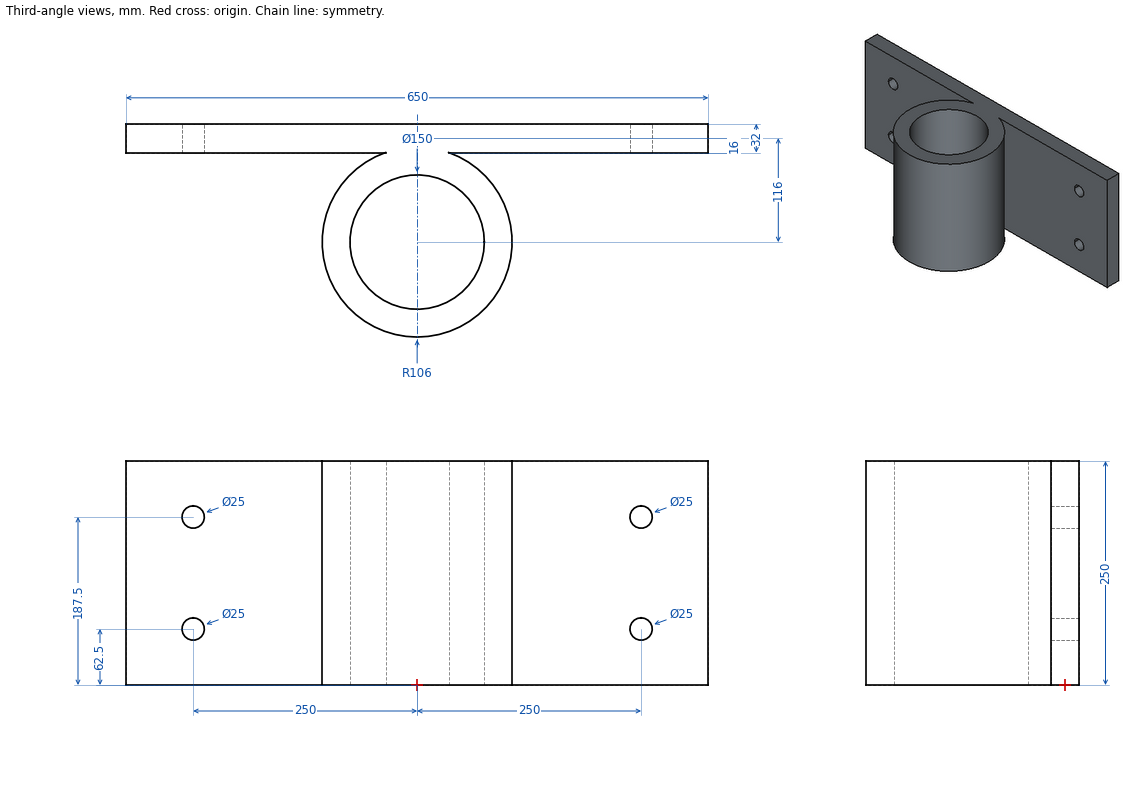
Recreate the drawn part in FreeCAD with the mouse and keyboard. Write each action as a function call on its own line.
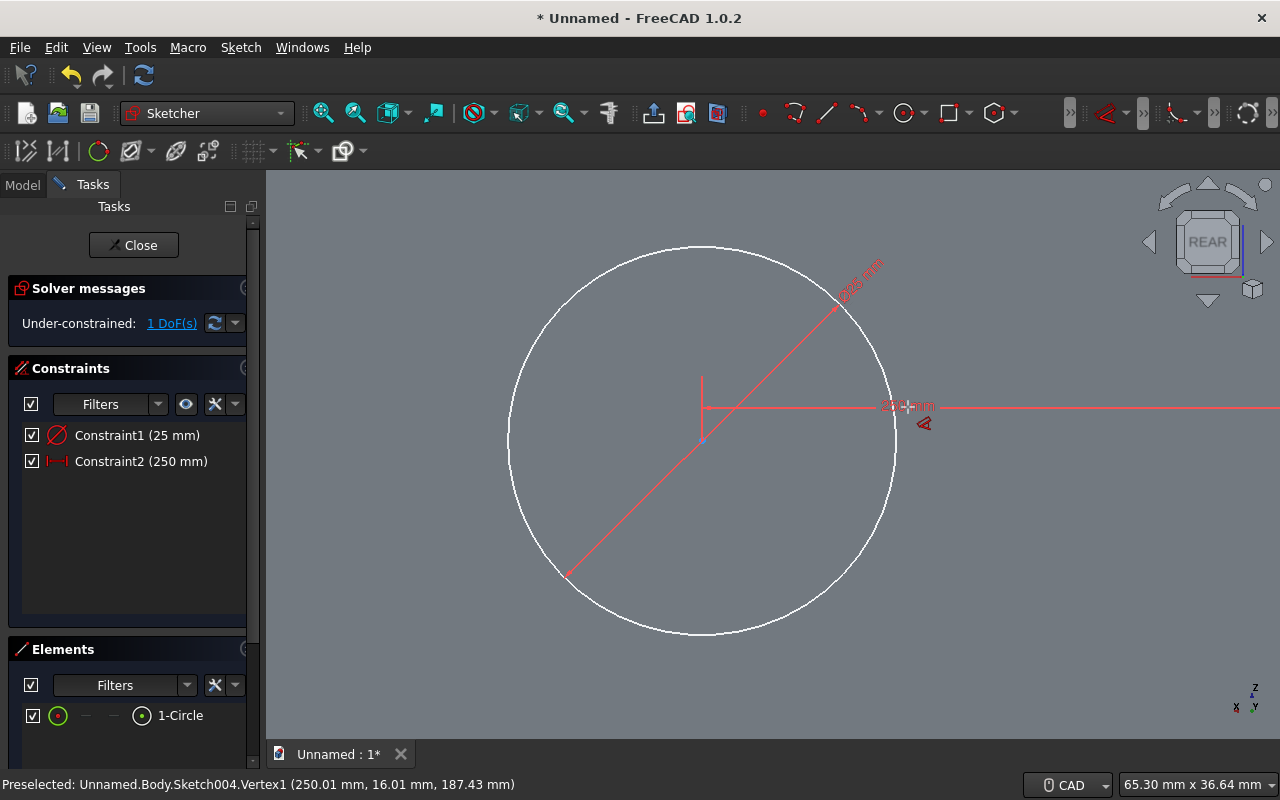
click(702, 441)
click(668, 576)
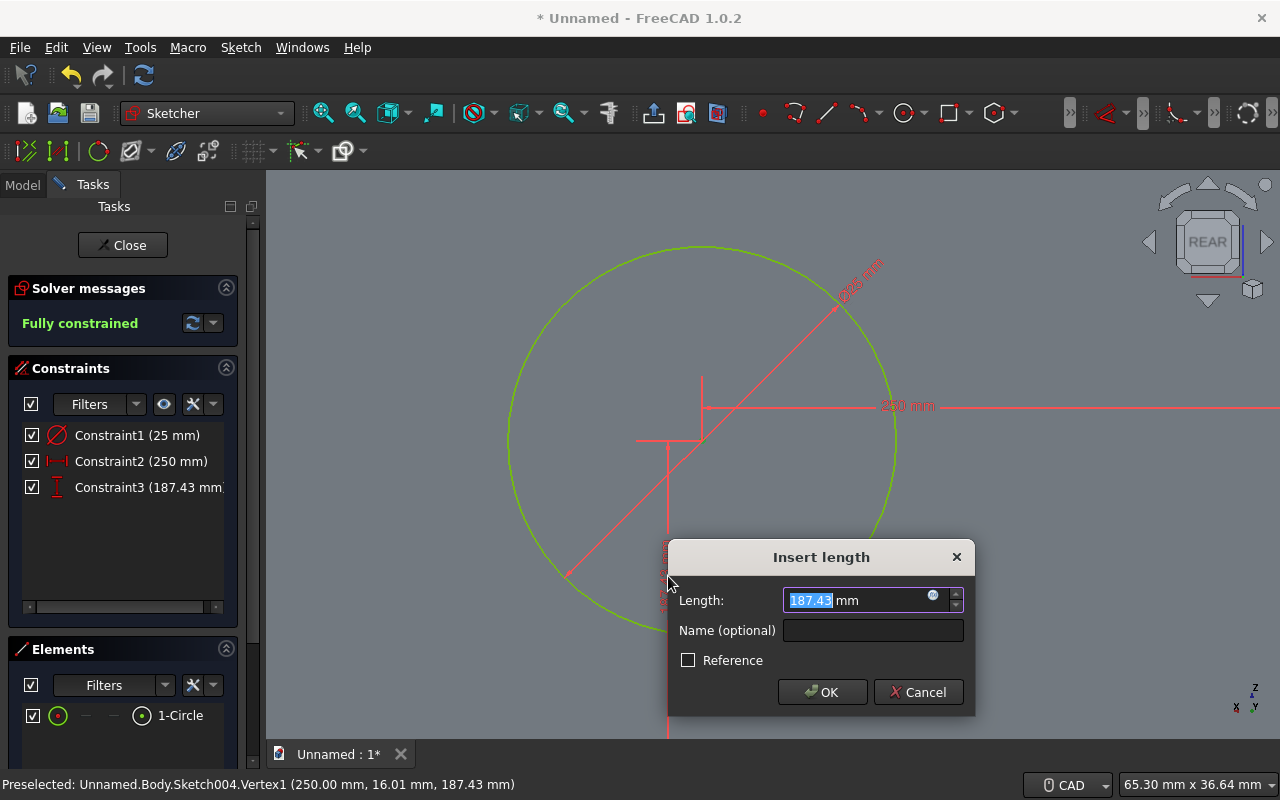
text(187.5)
key(Return)
key(Escape)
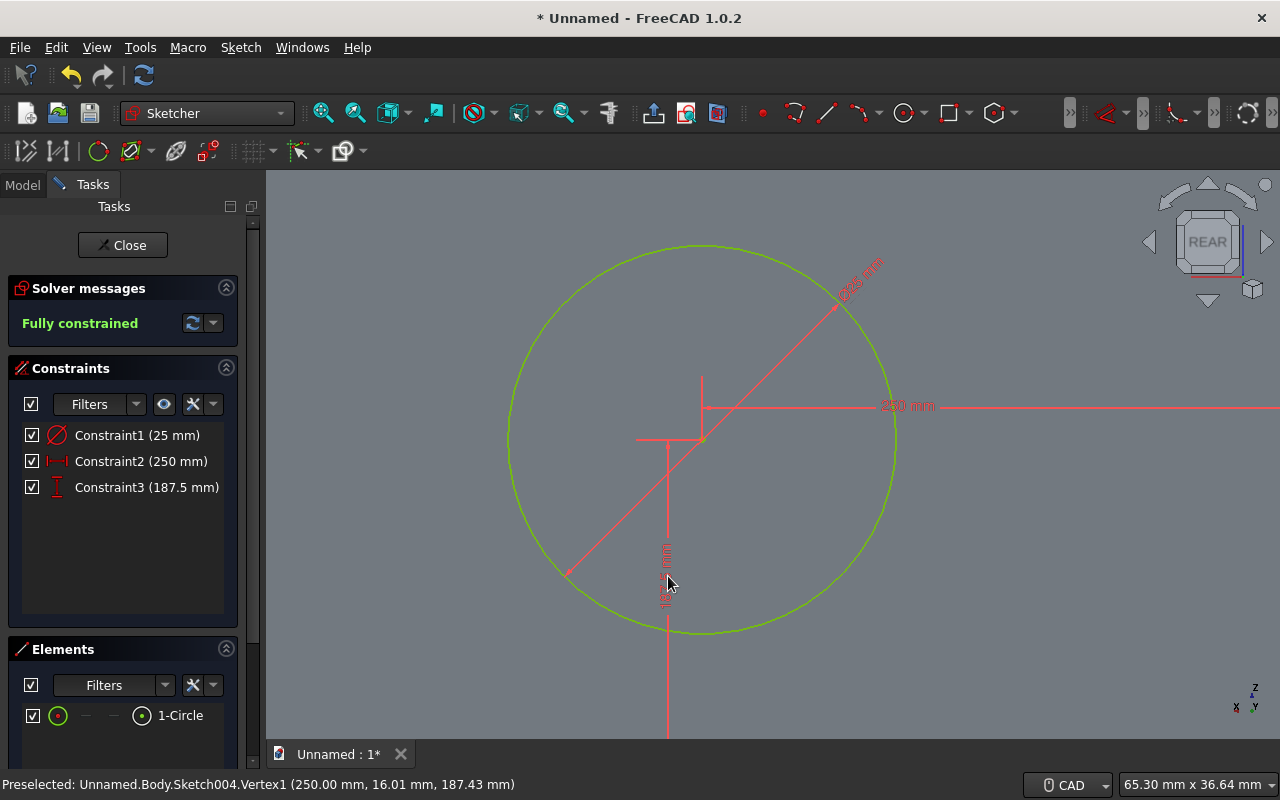
click(123, 245)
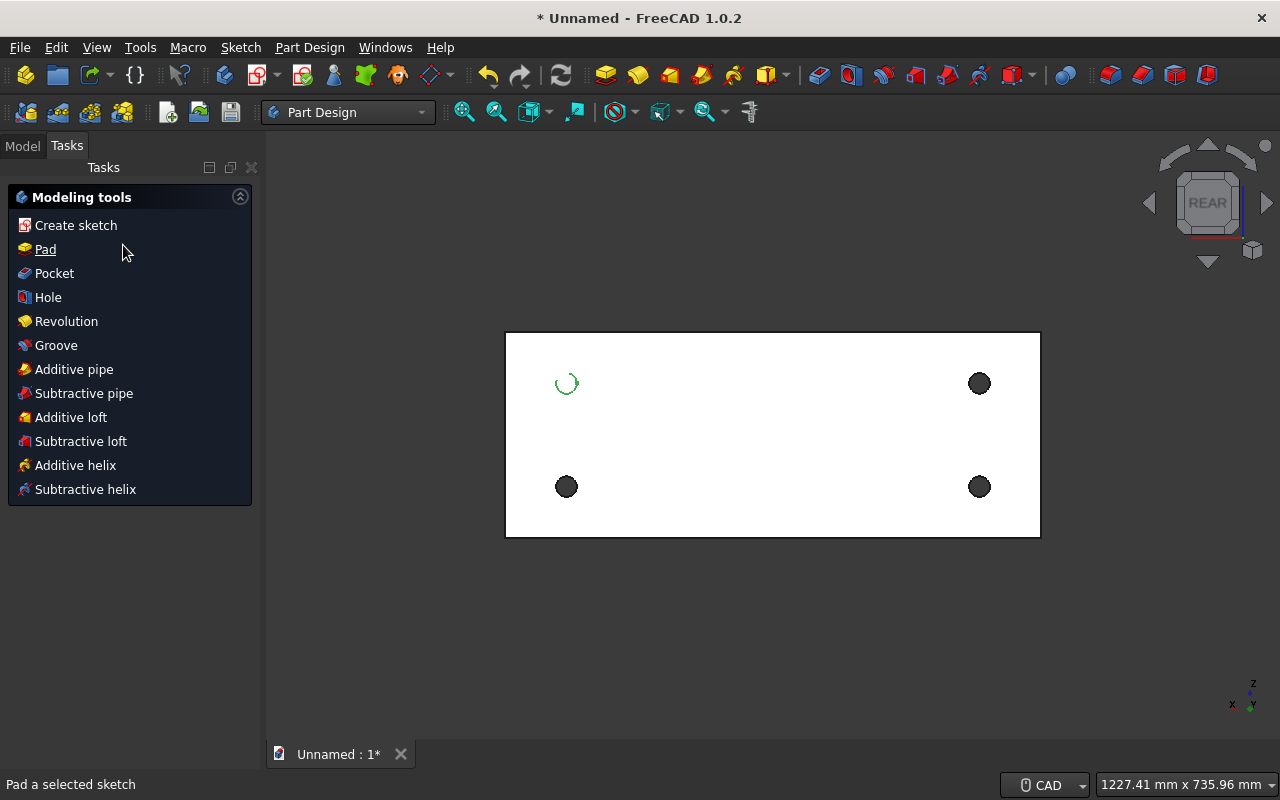
click(820, 76)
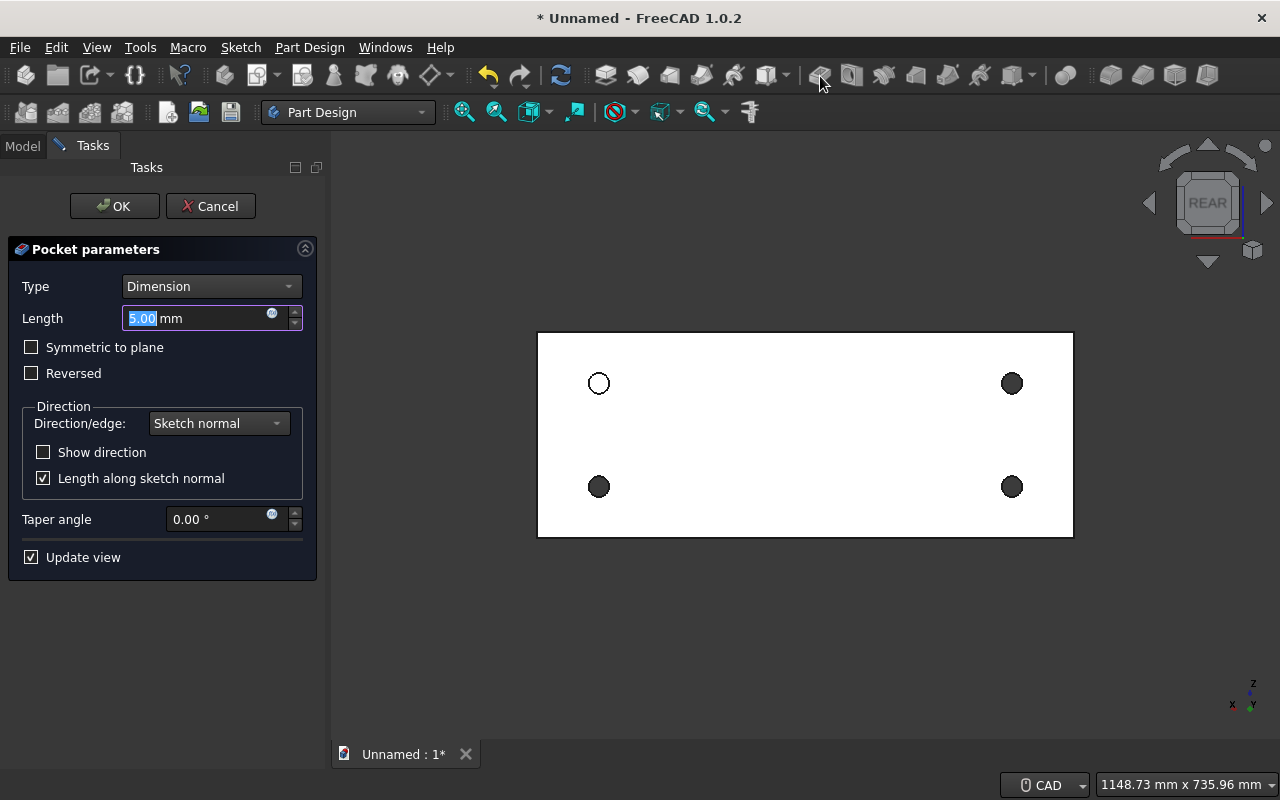
click(212, 286)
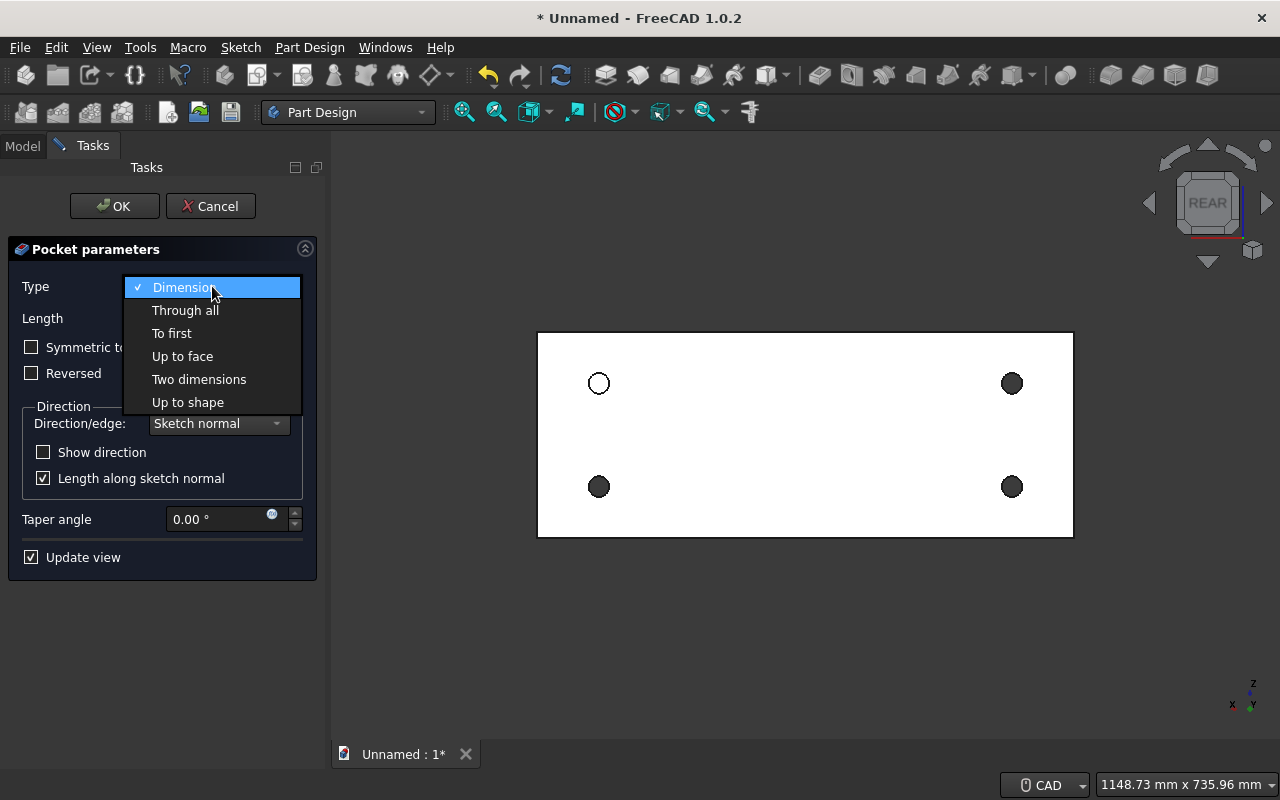
click(212, 334)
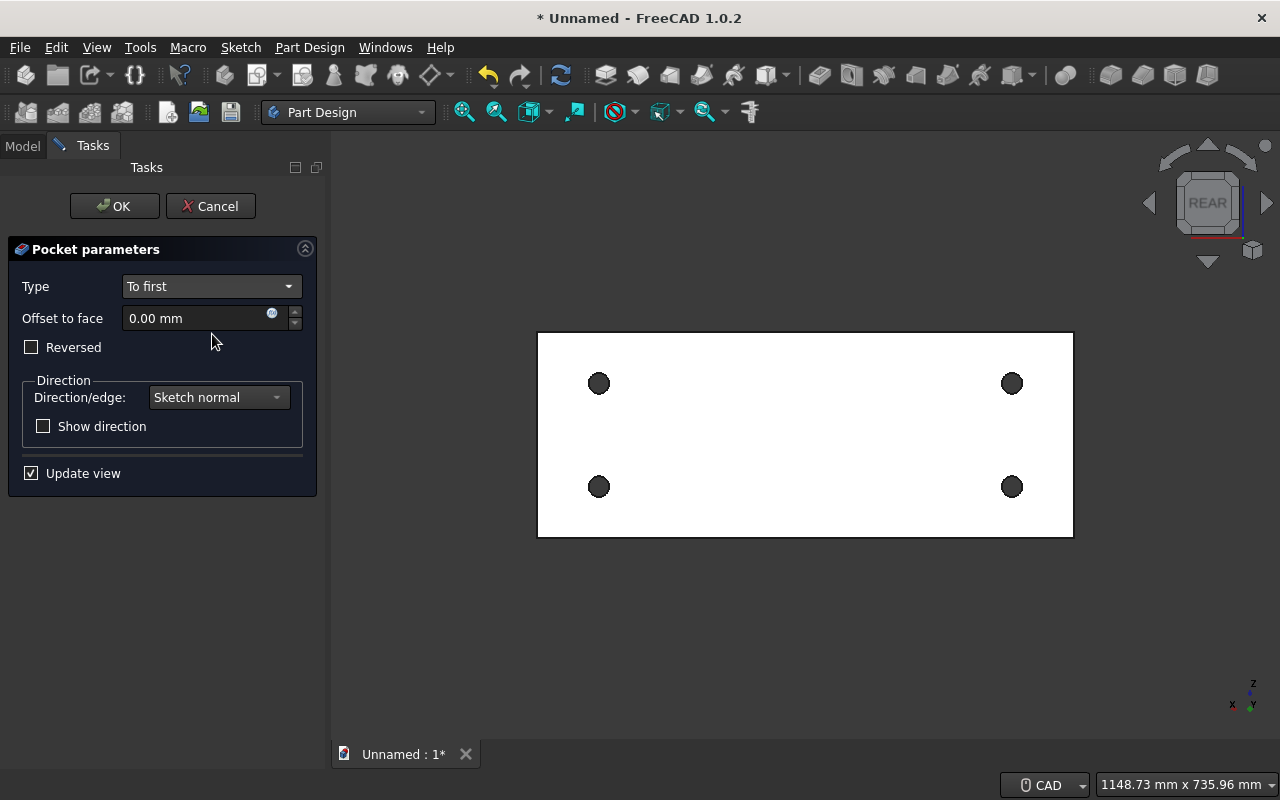
click(115, 206)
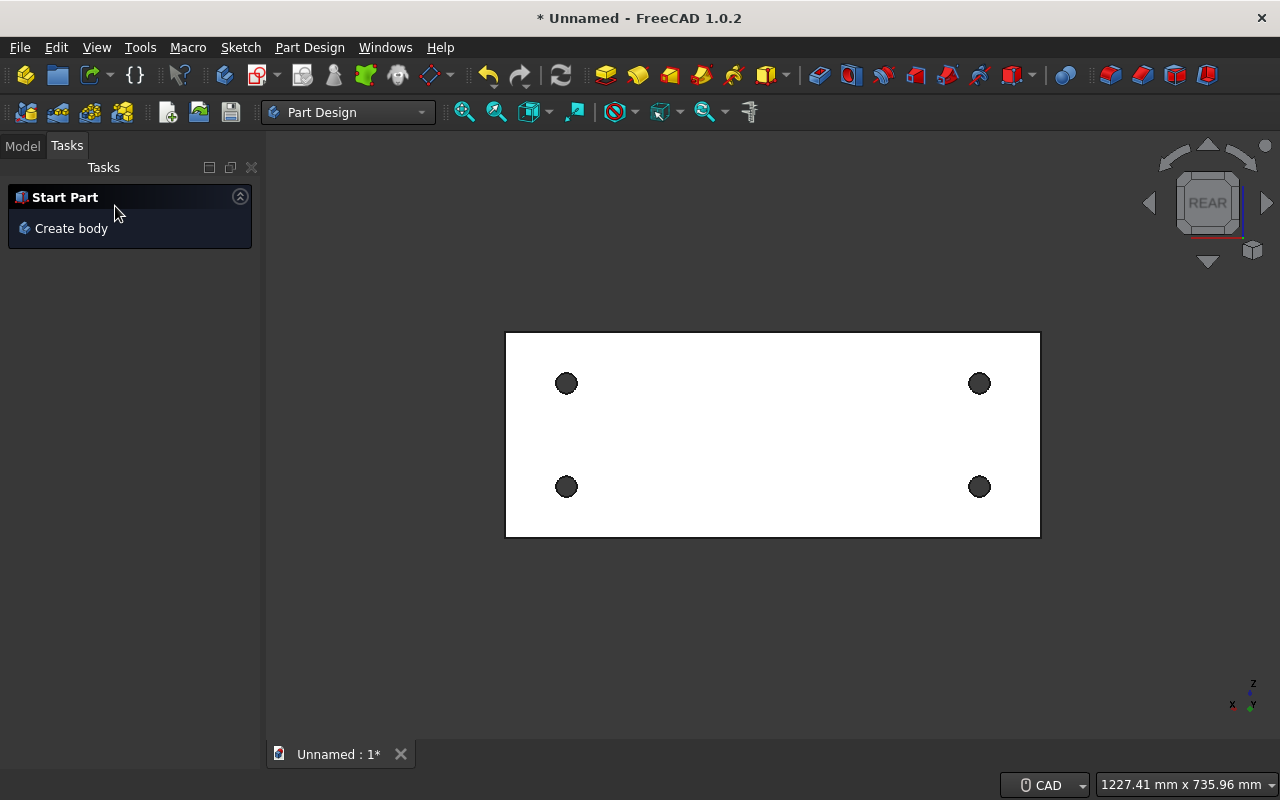
key(0)